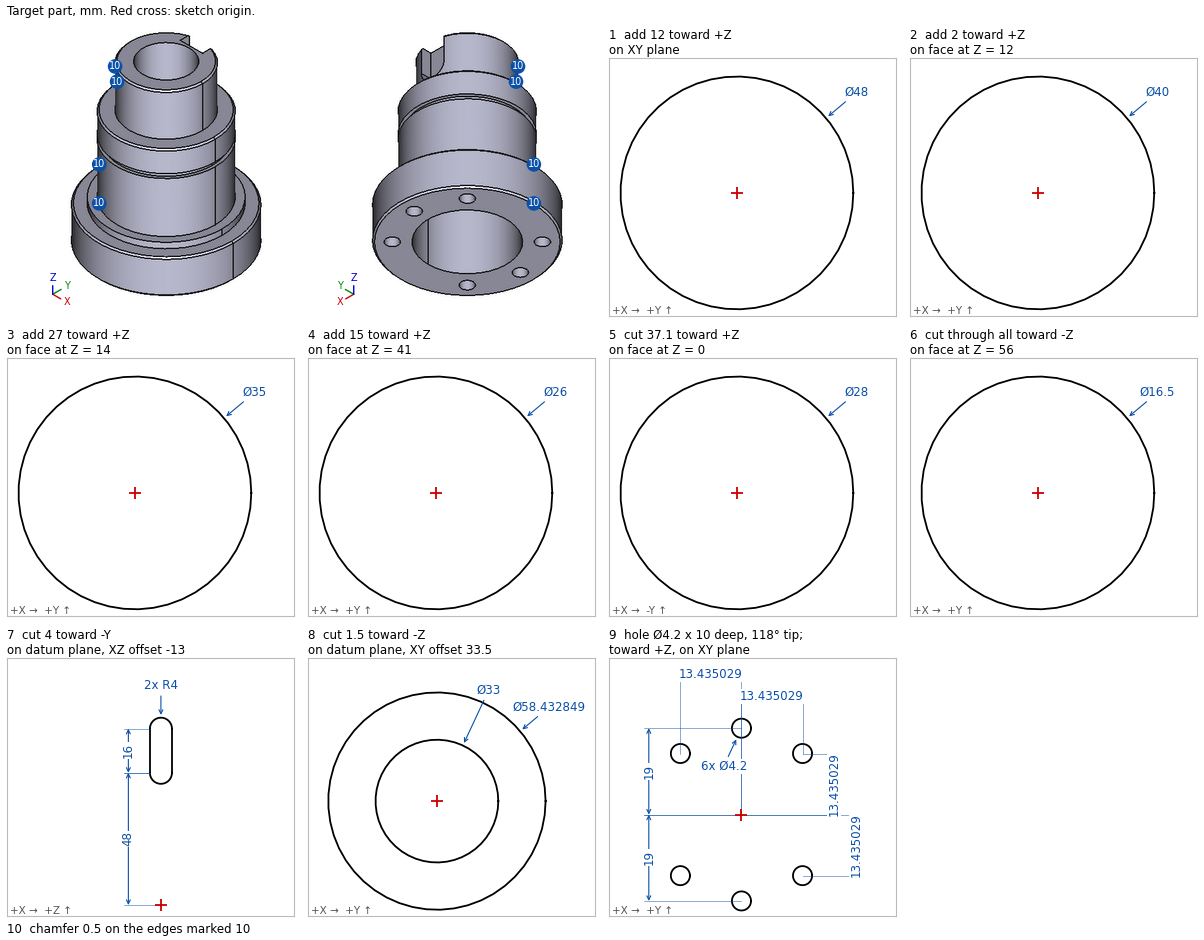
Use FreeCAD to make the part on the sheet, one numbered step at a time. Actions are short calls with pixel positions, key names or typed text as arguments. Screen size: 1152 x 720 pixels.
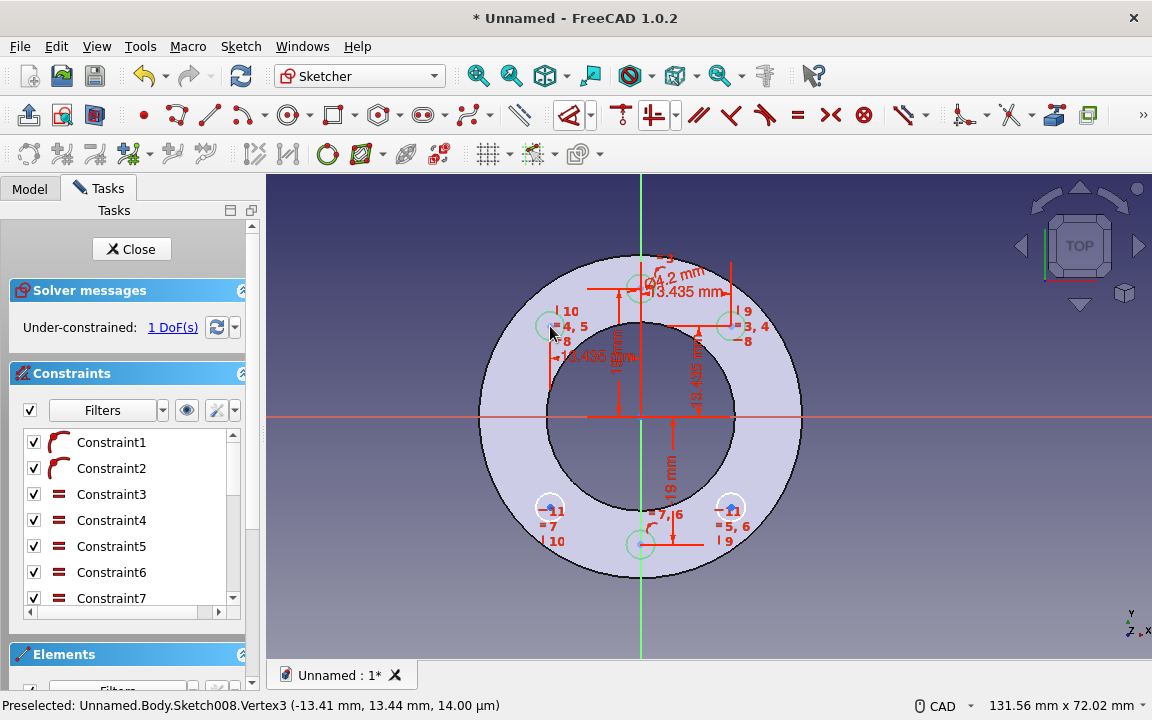
click(731, 507)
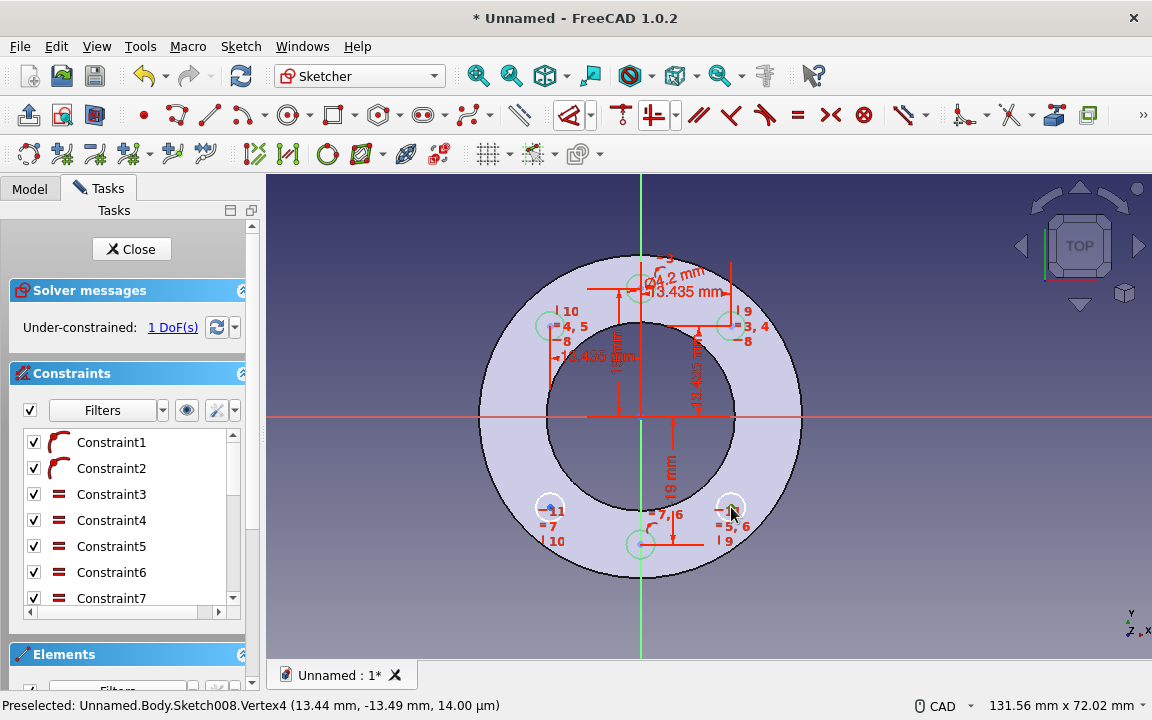
key(i)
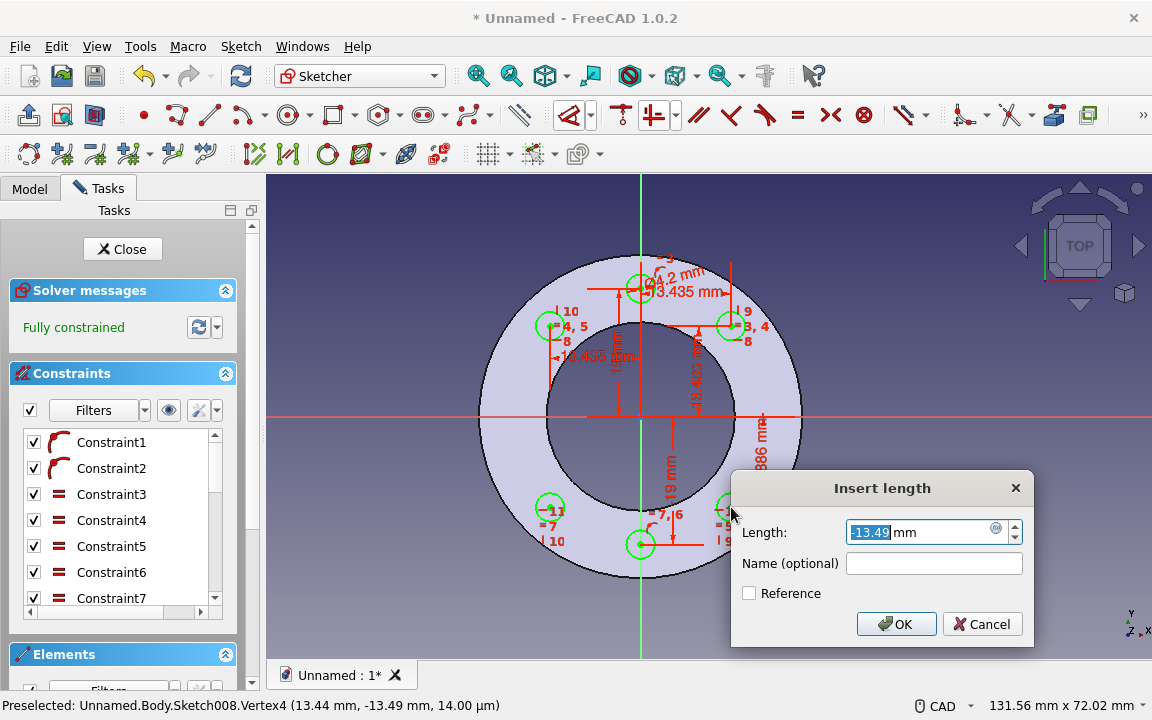
text(-13.435029)
key(Return)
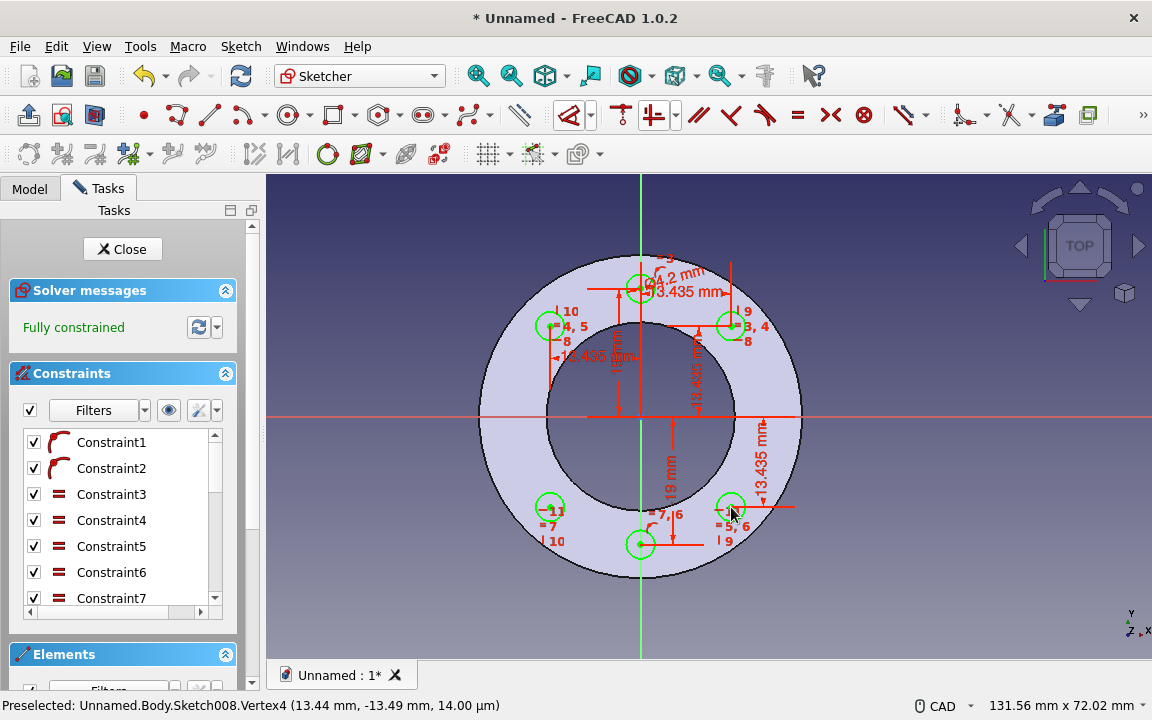
click(123, 249)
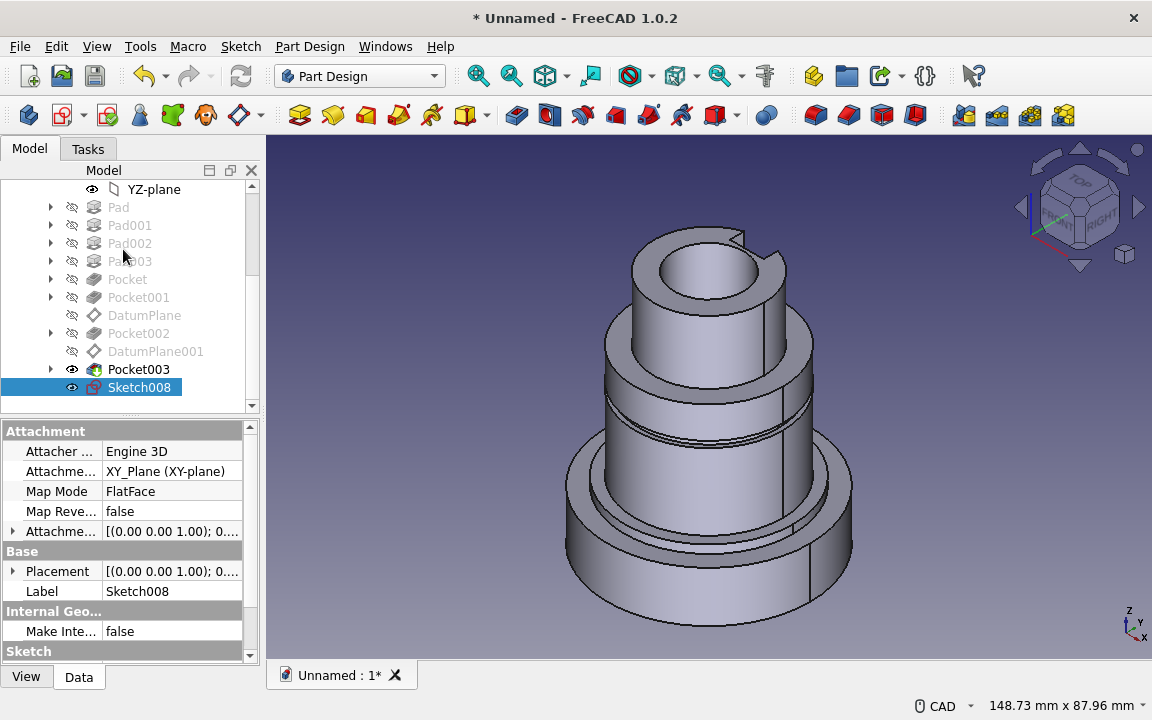
click(550, 116)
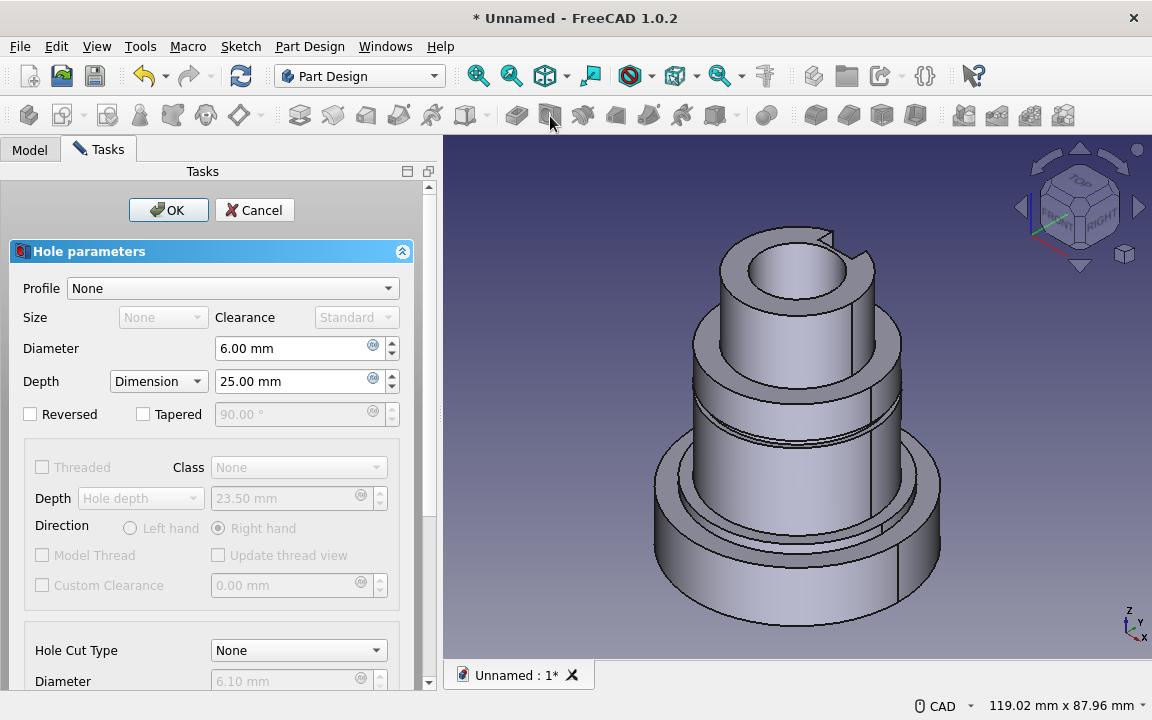
triple_click(300, 348)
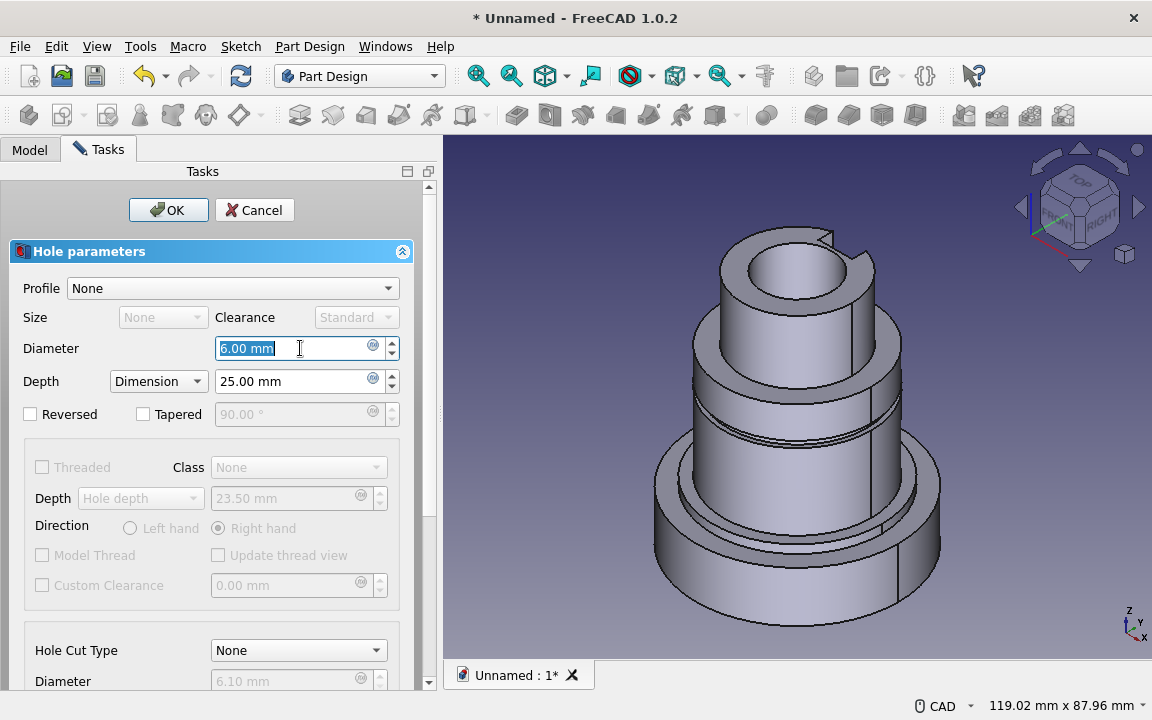
text(4.2)
key(Tab)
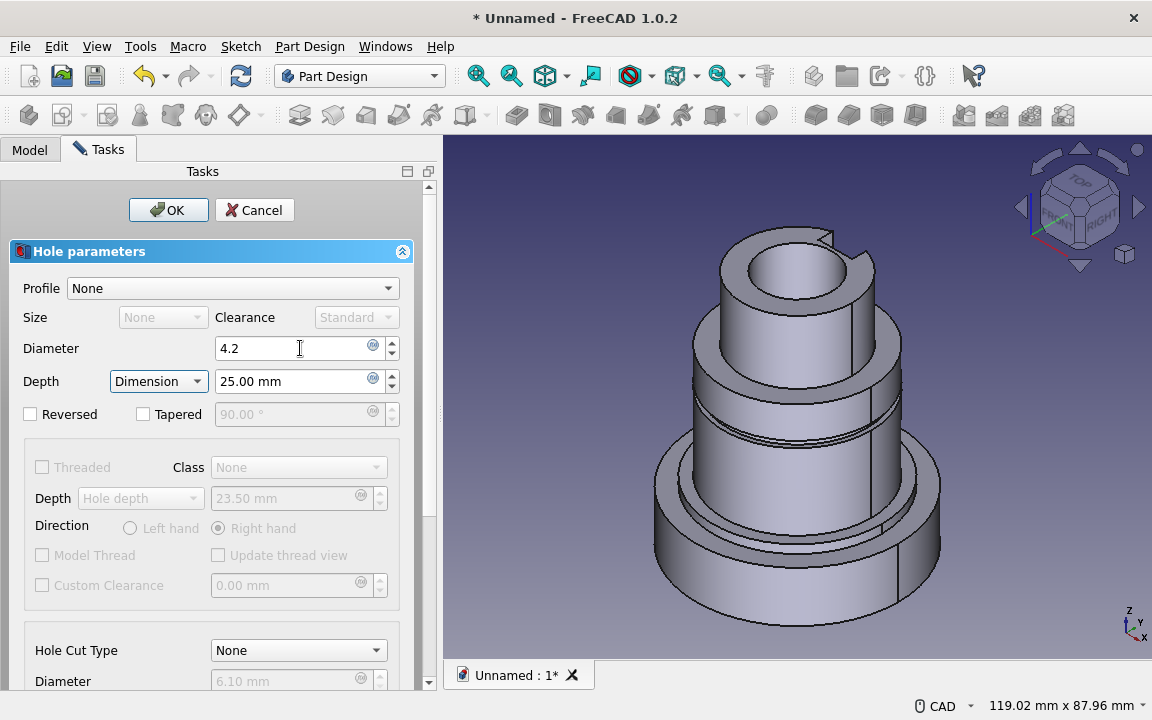
triple_click(300, 382)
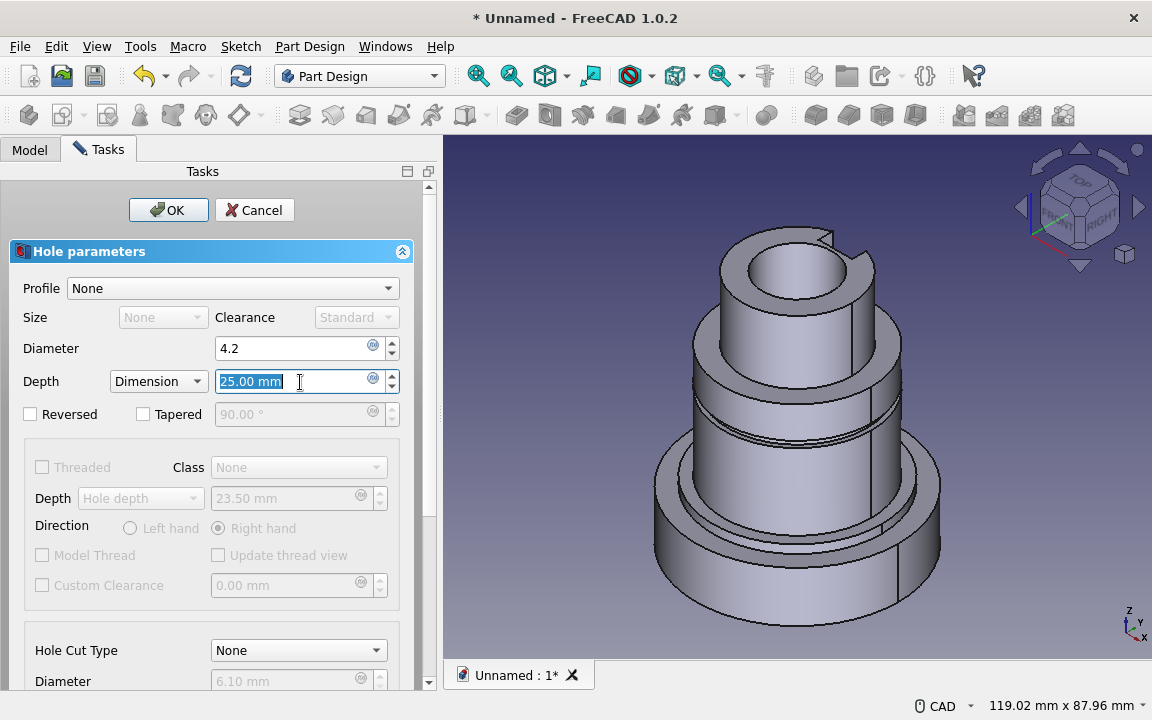
text(10)
key(Tab)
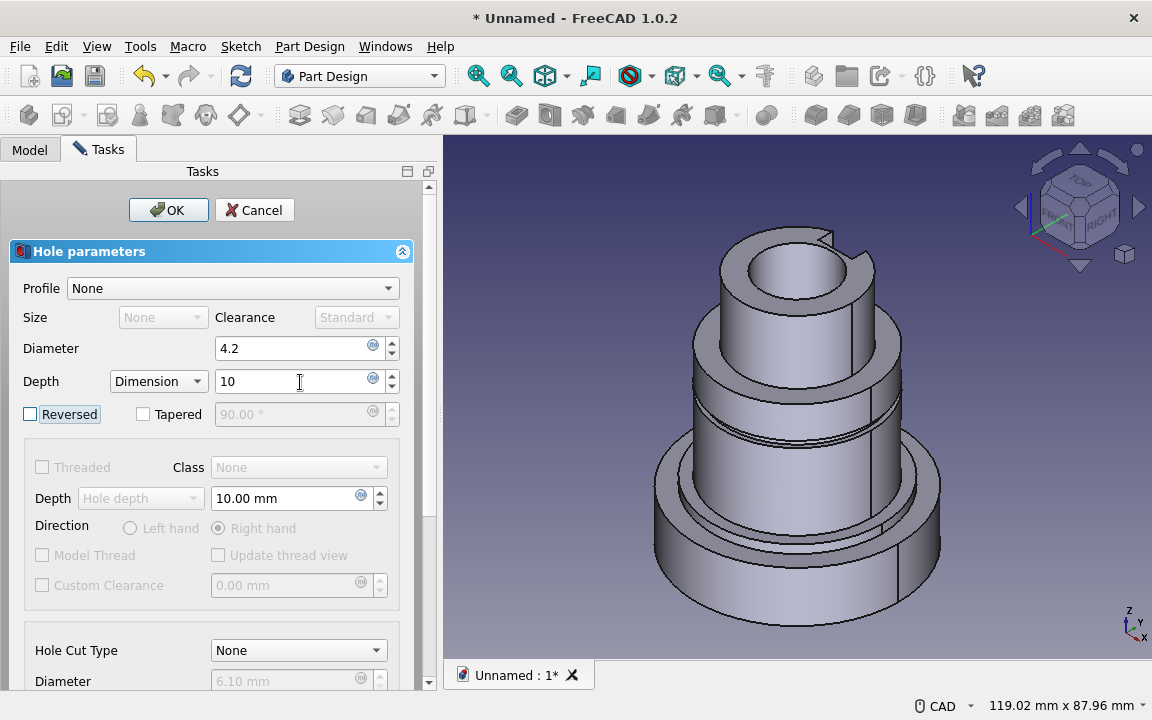
click(31, 414)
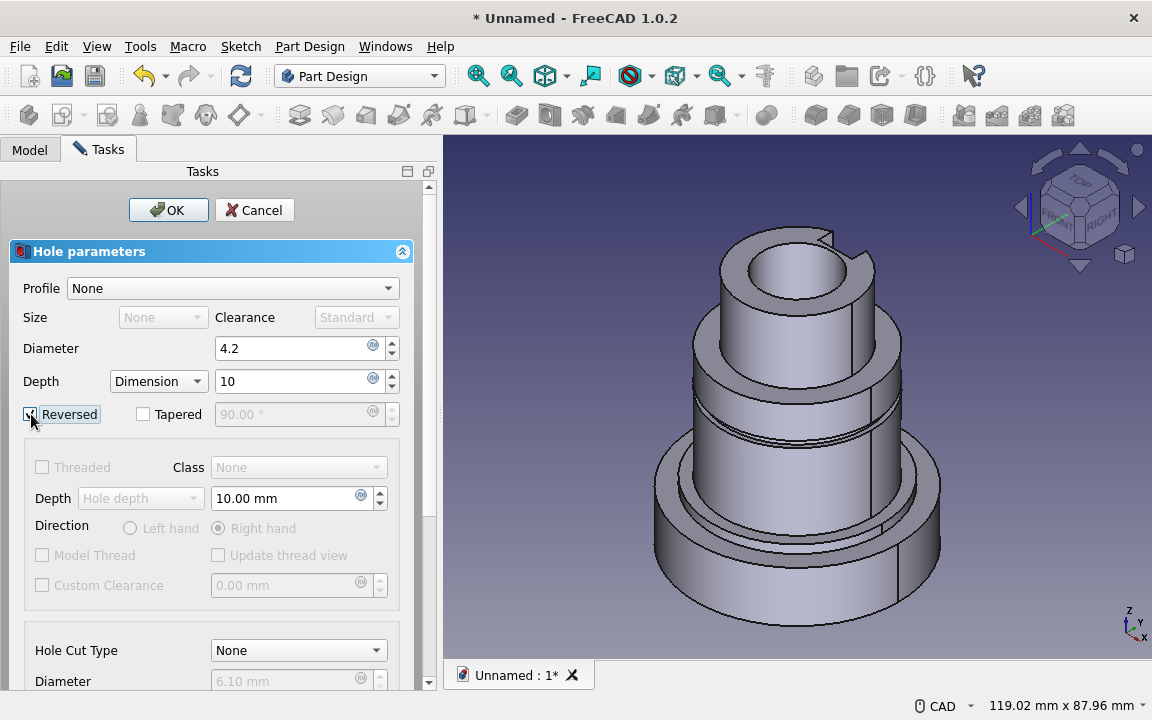
click(169, 210)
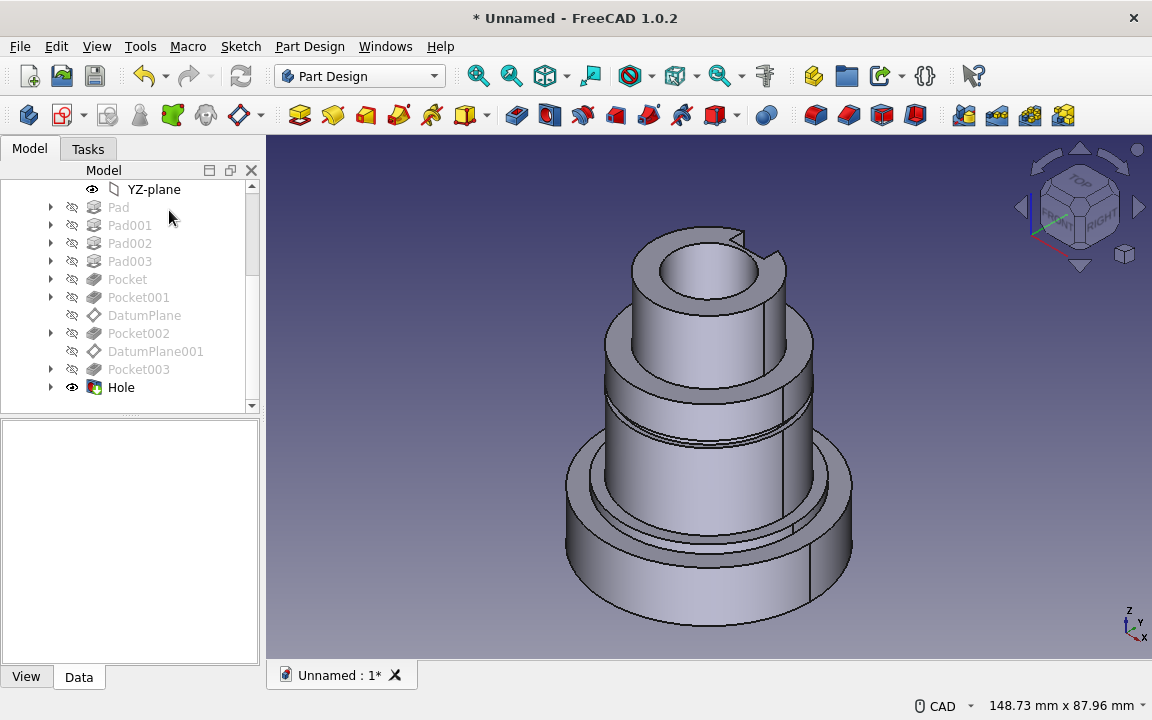
click(616, 371)